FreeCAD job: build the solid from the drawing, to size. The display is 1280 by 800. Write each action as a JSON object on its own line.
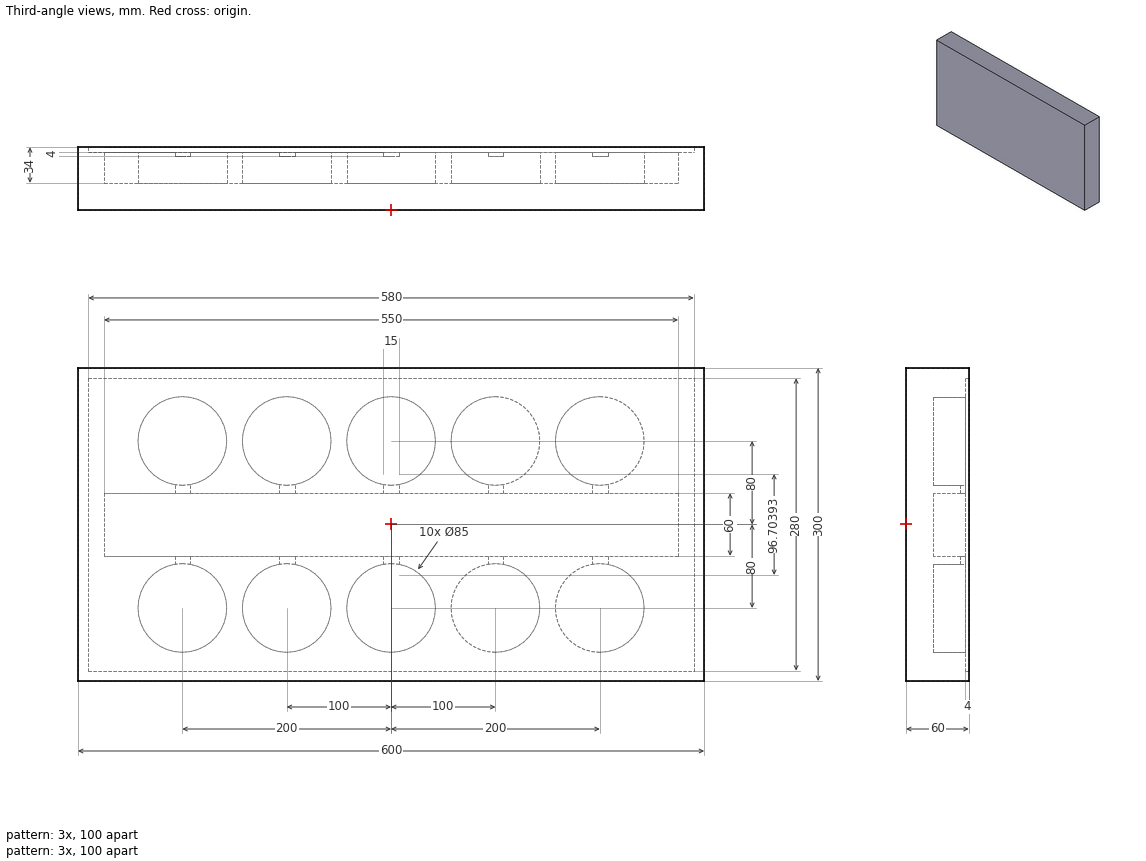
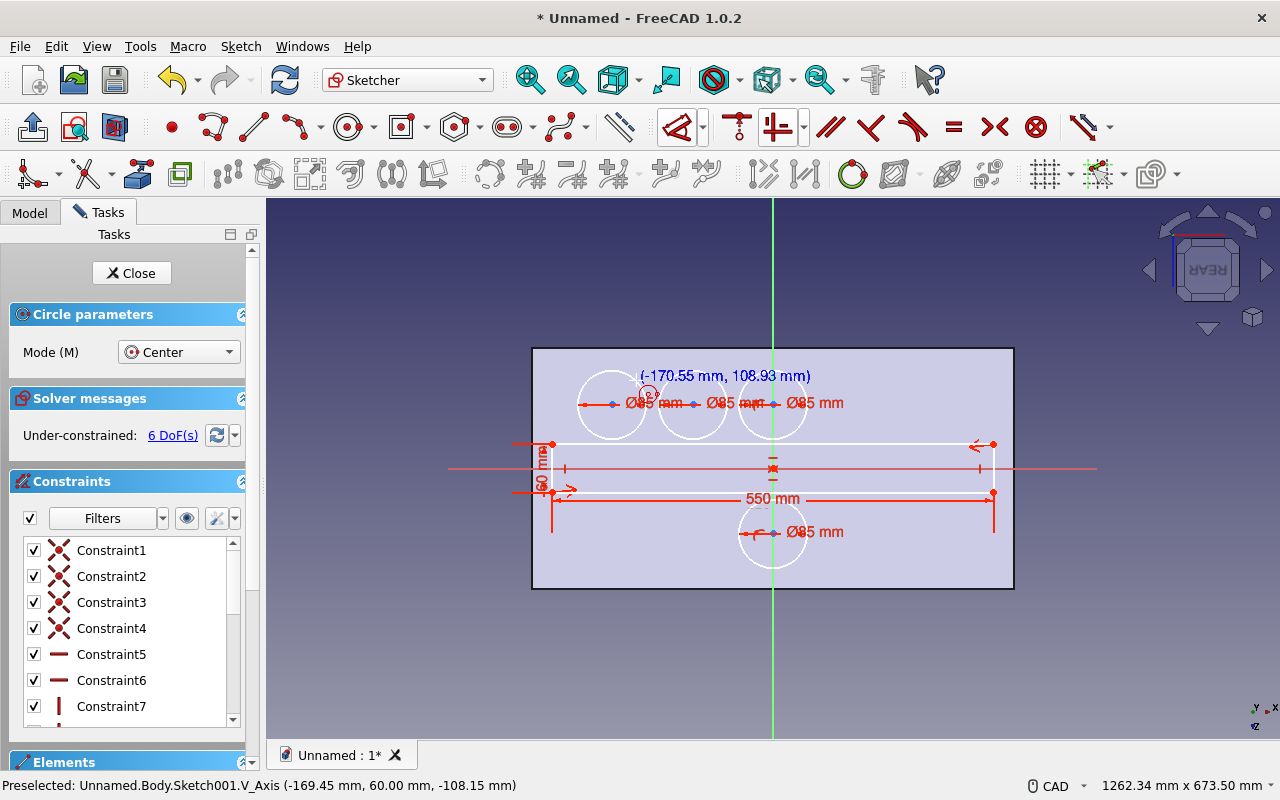
{"action": "left_click", "coordinate": [934, 404]}
{"action": "mouse_move", "coordinate": [958, 380]}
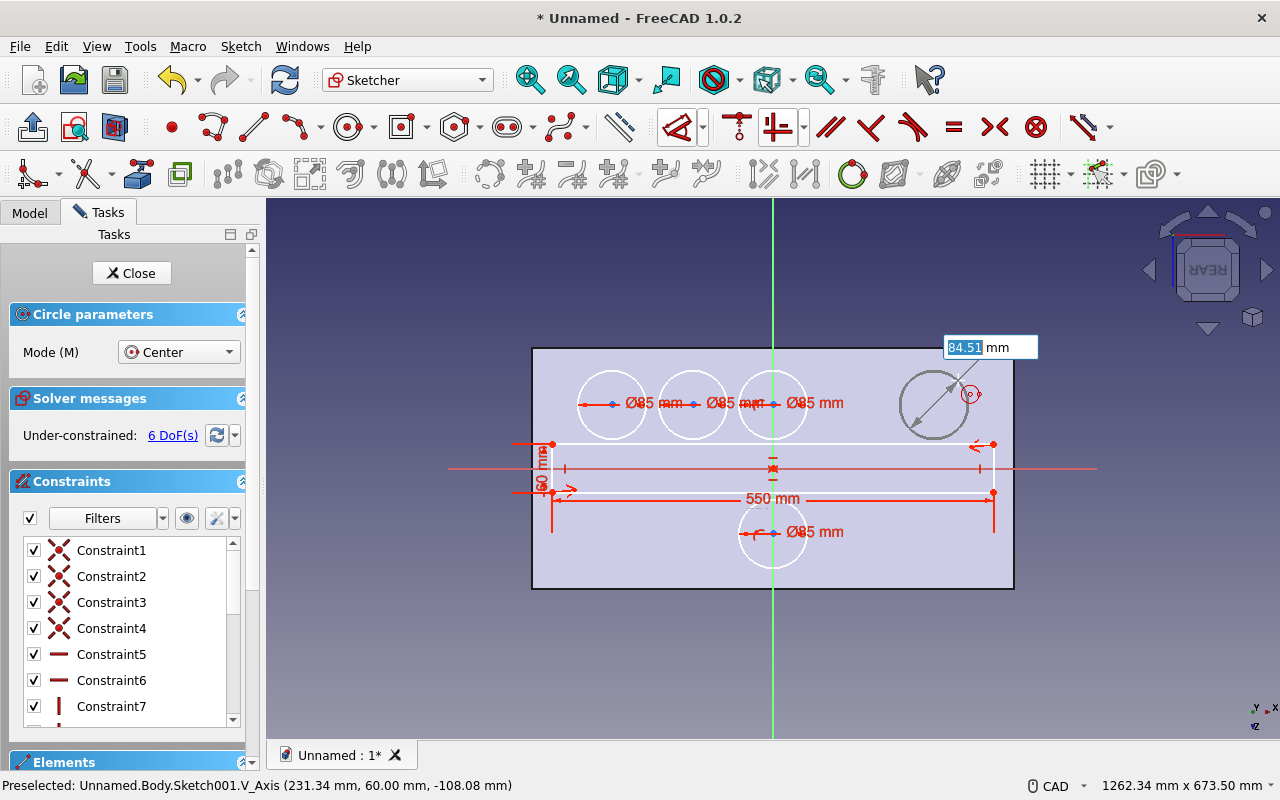
{"action": "type", "text": "85"}
{"action": "key", "text": "Return"}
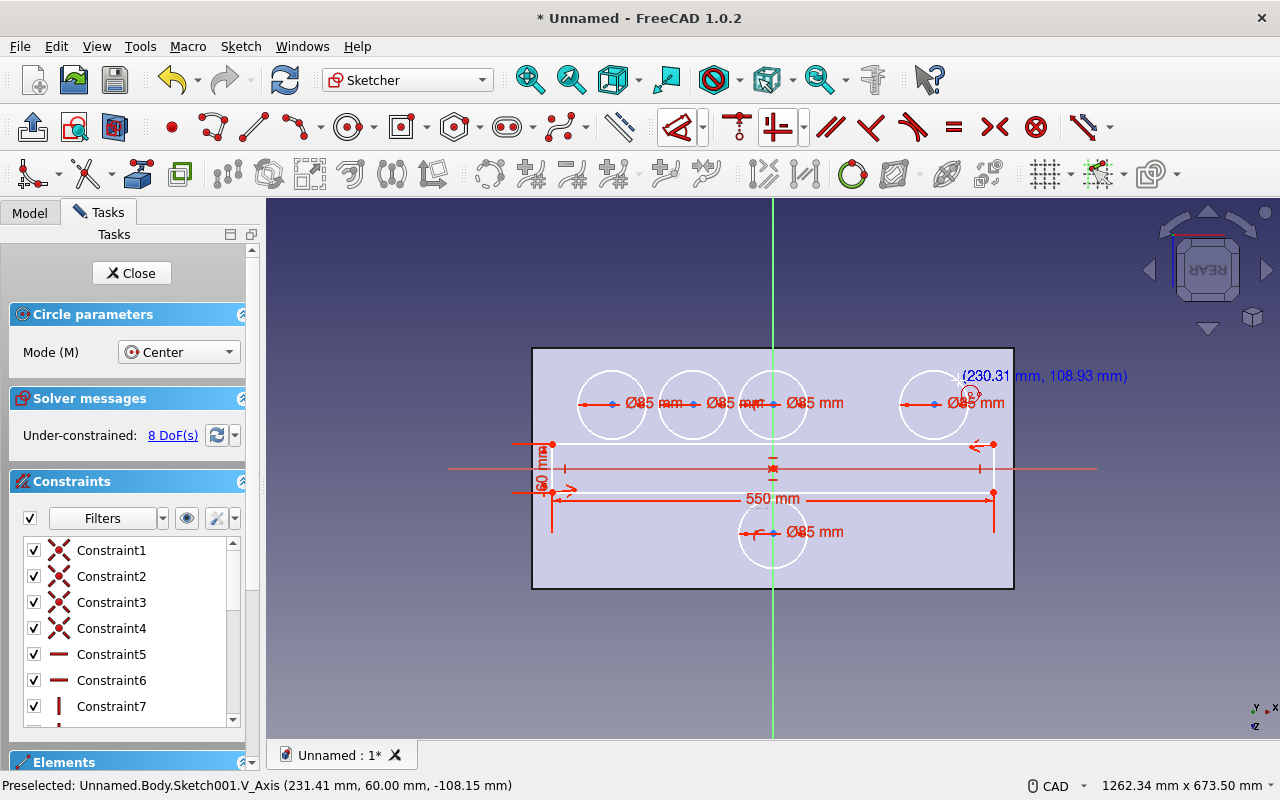
{"action": "left_click", "coordinate": [853, 404]}
{"action": "mouse_move", "coordinate": [877, 380]}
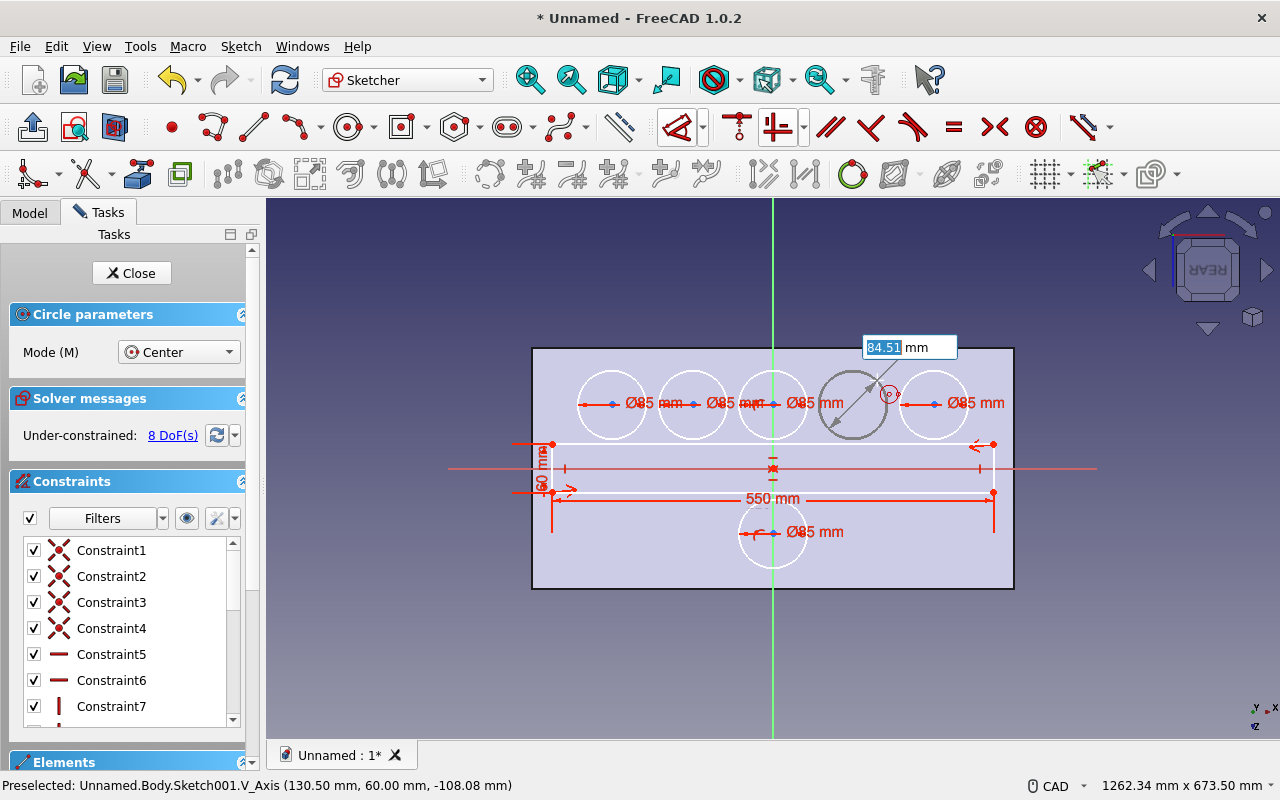
{"action": "type", "text": "85"}
{"action": "key", "text": "Return"}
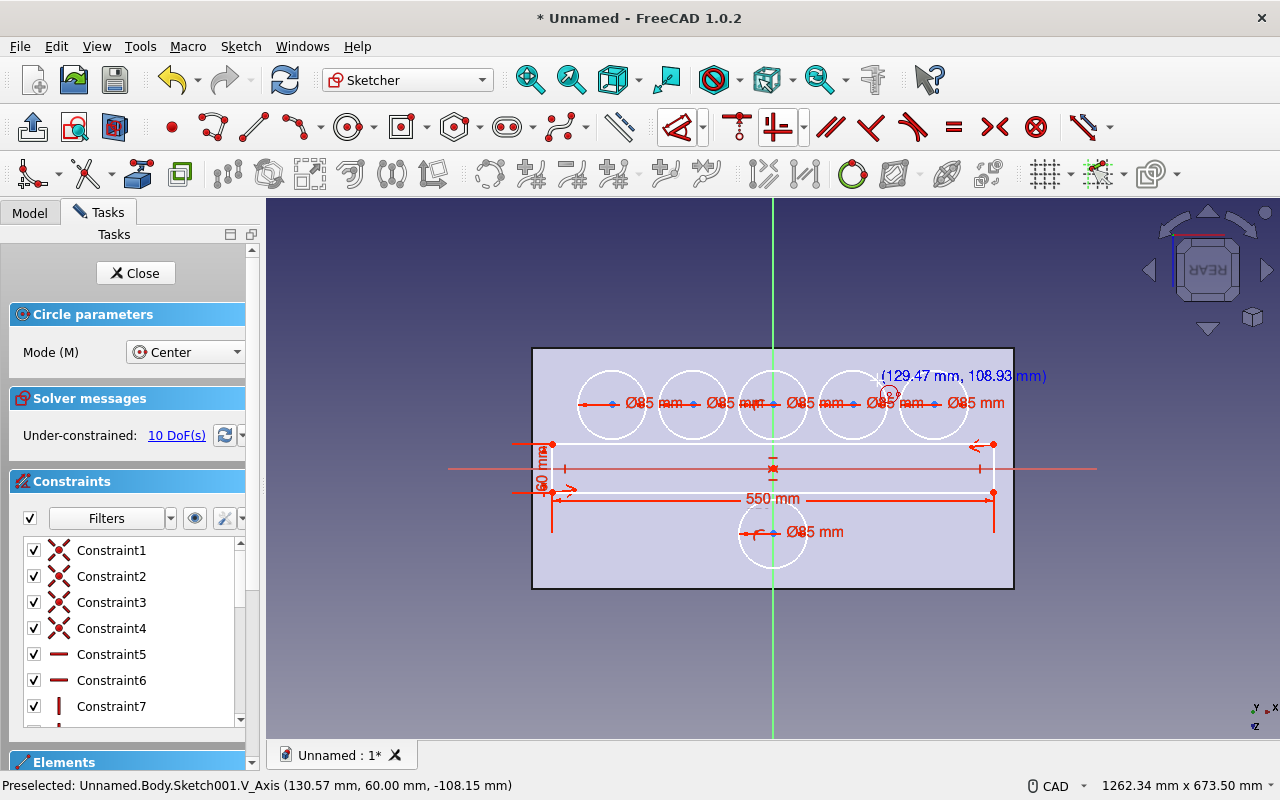
{"action": "left_click", "coordinate": [934, 533]}
{"action": "mouse_move", "coordinate": [958, 509]}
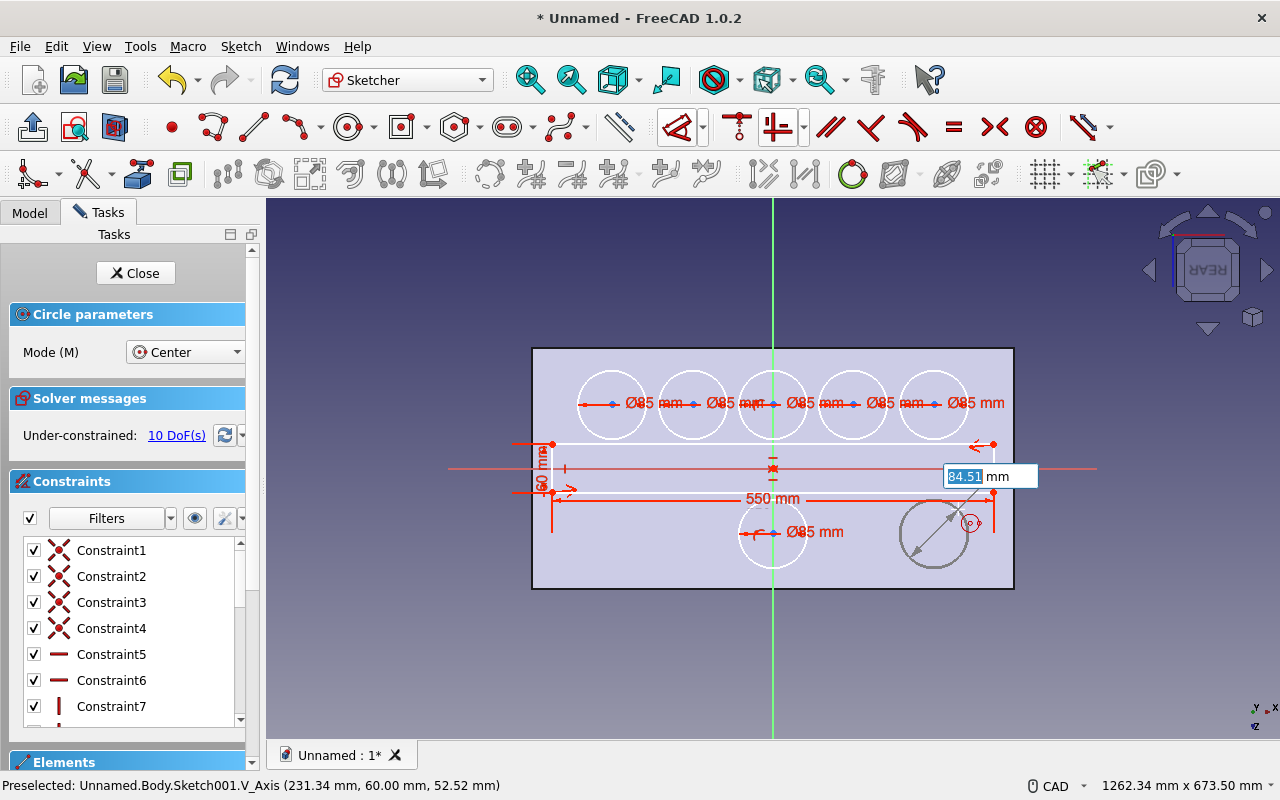
{"action": "type", "text": "85"}
{"action": "key", "text": "Return"}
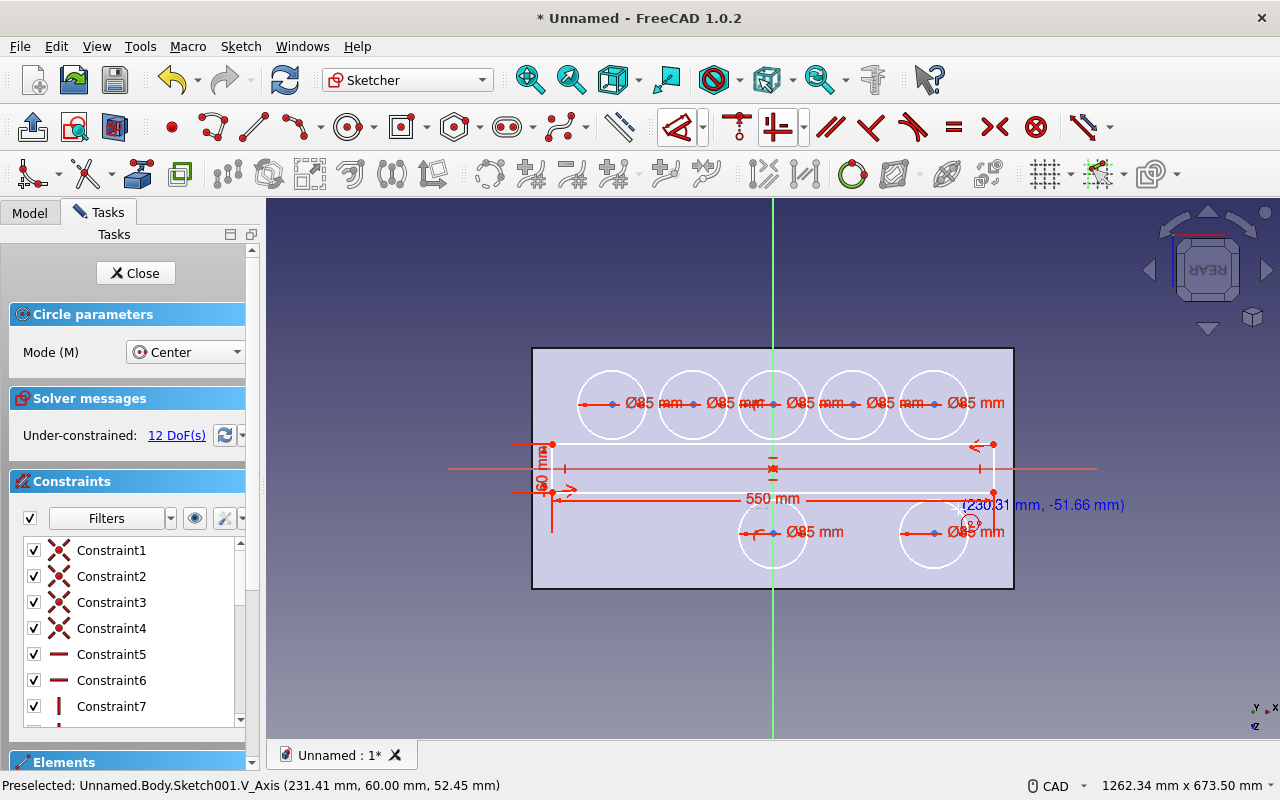
{"action": "left_click", "coordinate": [853, 533]}
{"action": "mouse_move", "coordinate": [877, 509]}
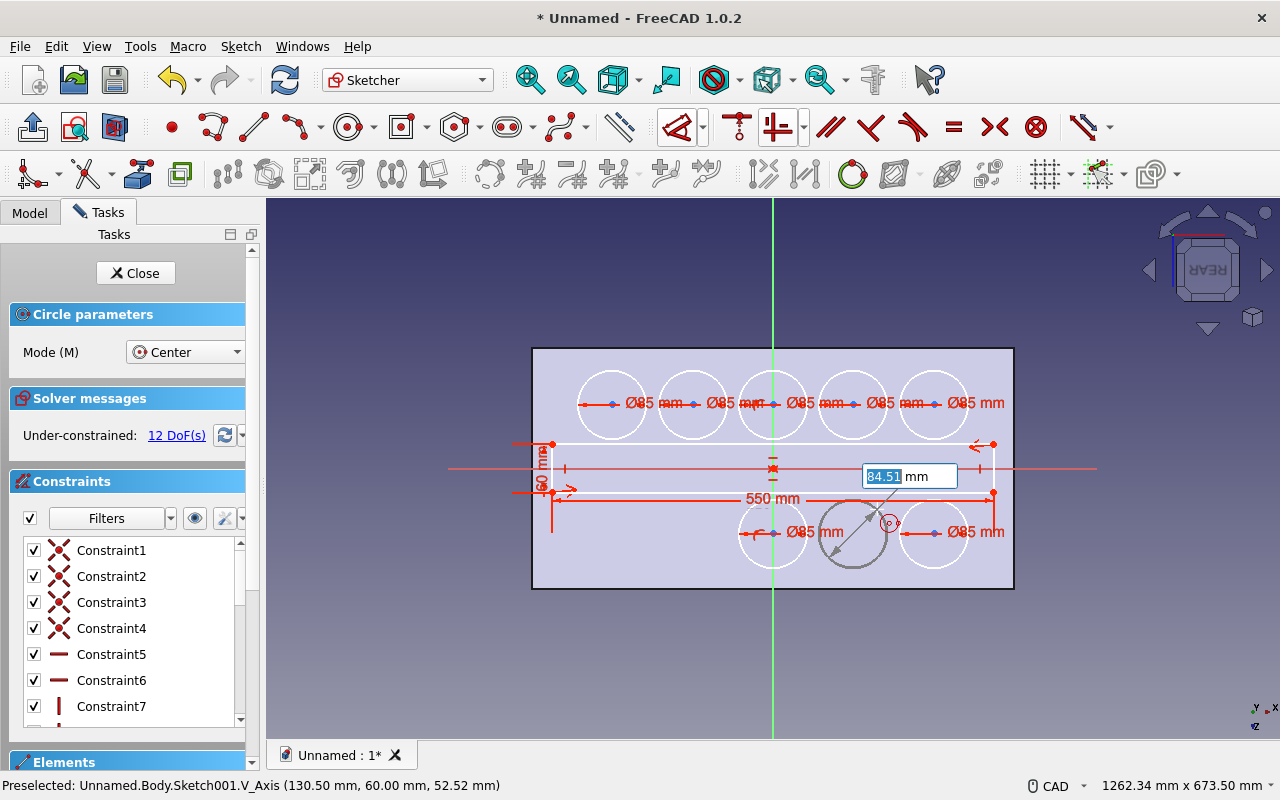
{"action": "type", "text": "85"}
{"action": "key", "text": "Return"}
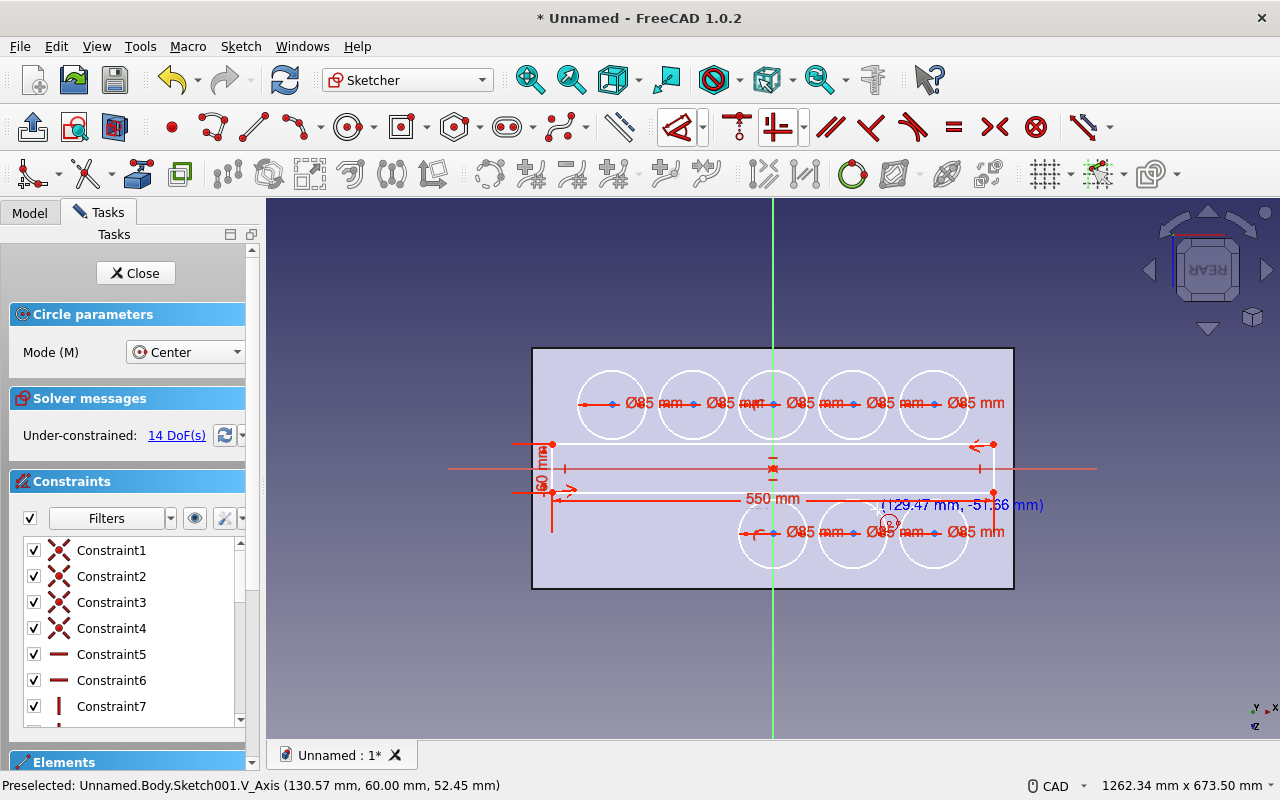
{"action": "left_click", "coordinate": [693, 533]}
{"action": "mouse_move", "coordinate": [717, 509]}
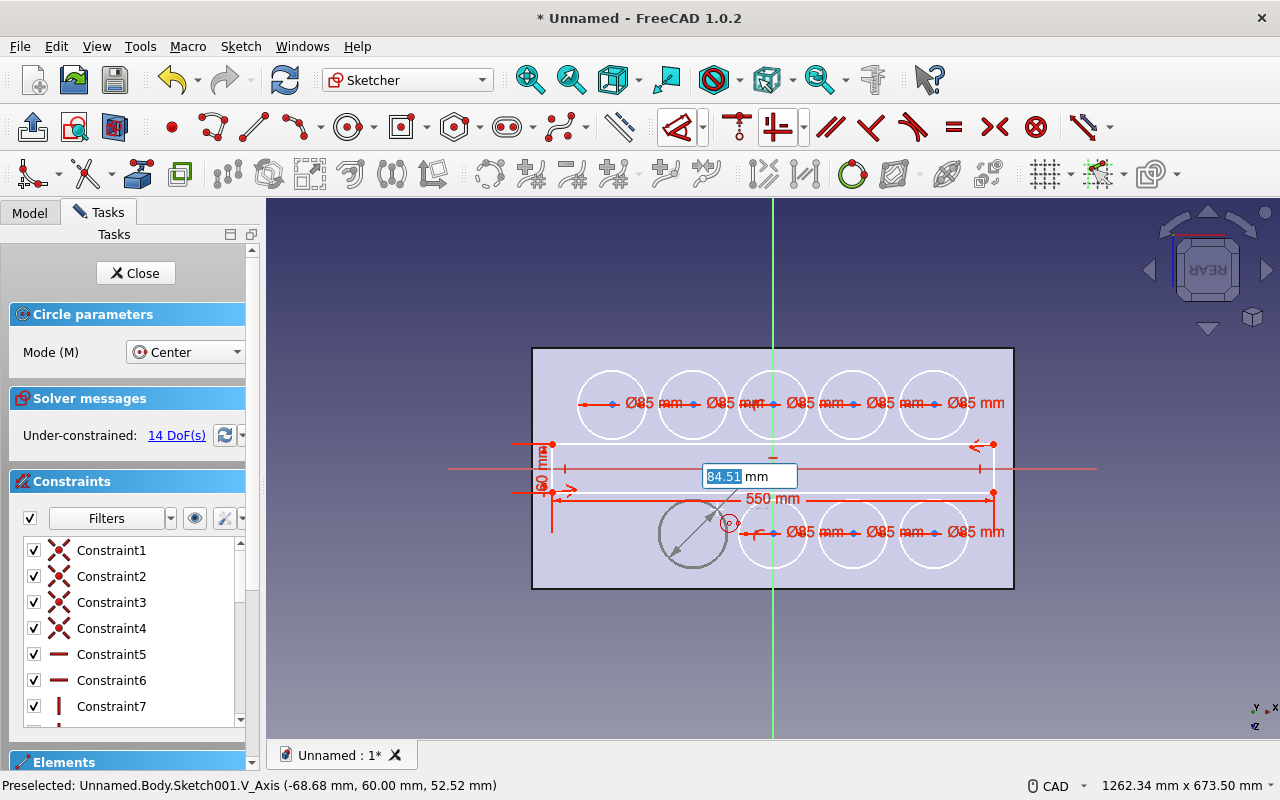
{"action": "type", "text": "85"}
{"action": "key", "text": "Return"}